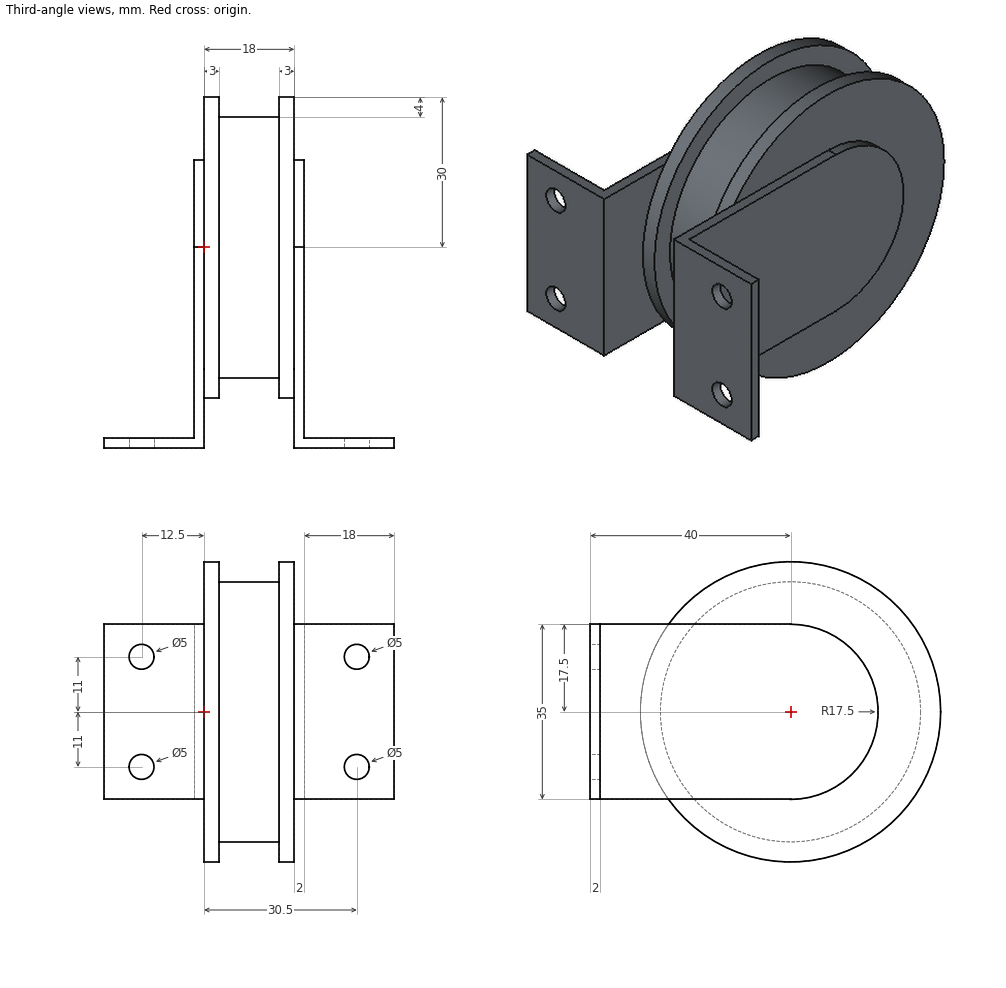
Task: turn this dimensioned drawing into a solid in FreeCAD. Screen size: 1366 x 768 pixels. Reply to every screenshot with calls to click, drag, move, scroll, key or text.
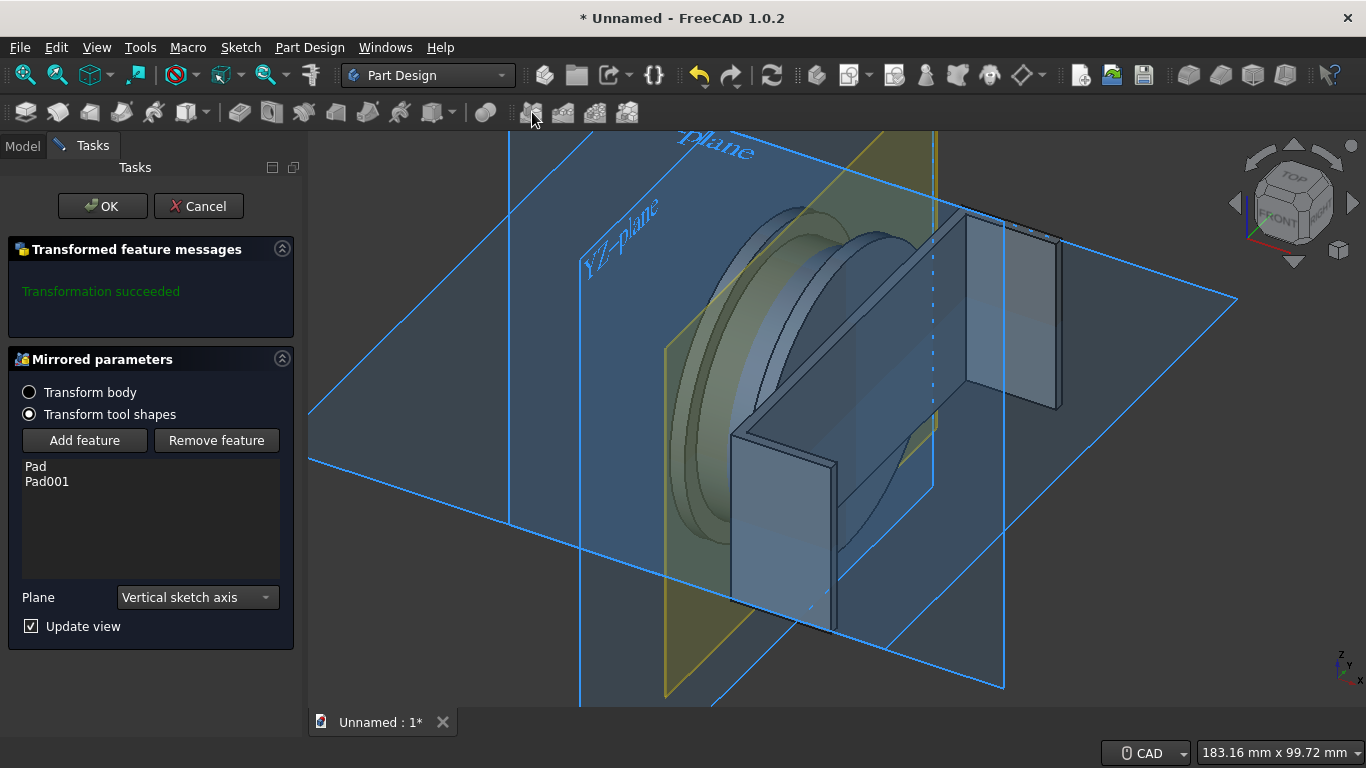
click(198, 598)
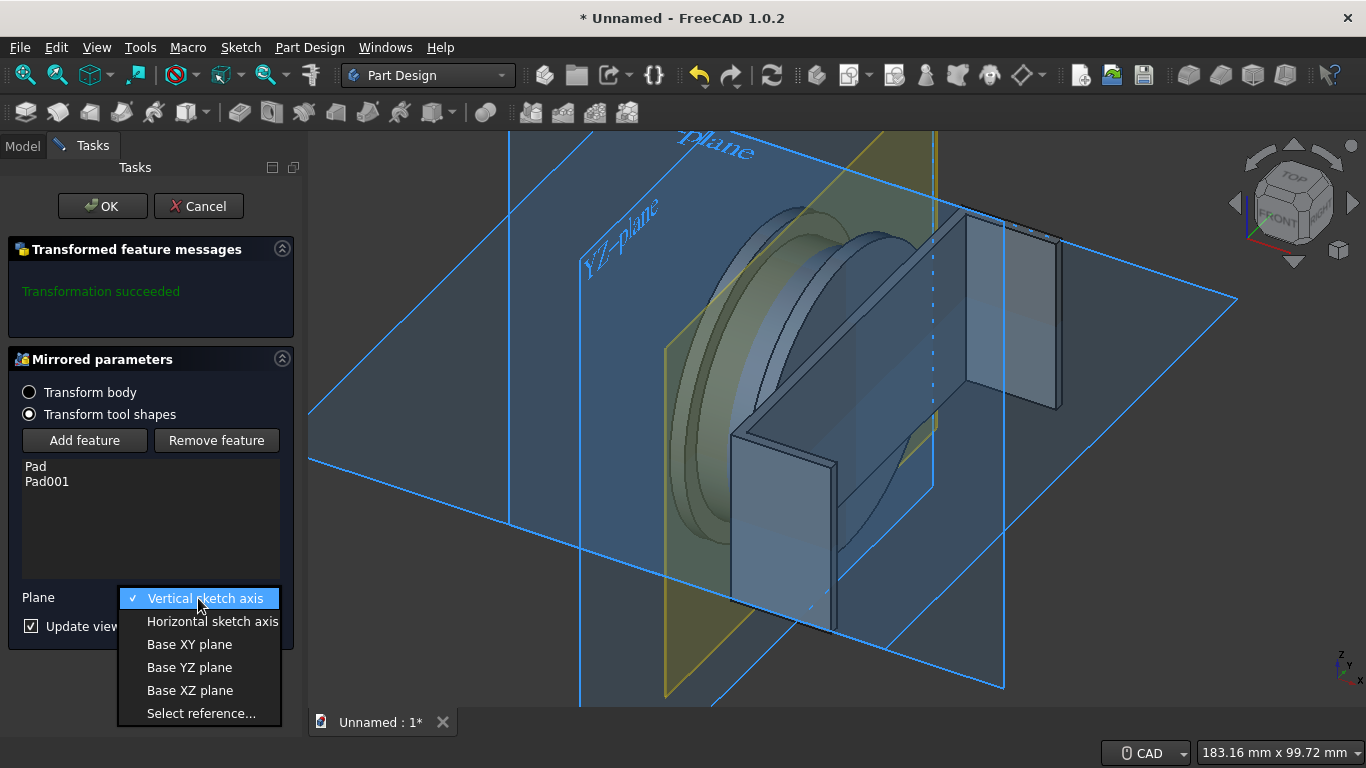
click(198, 714)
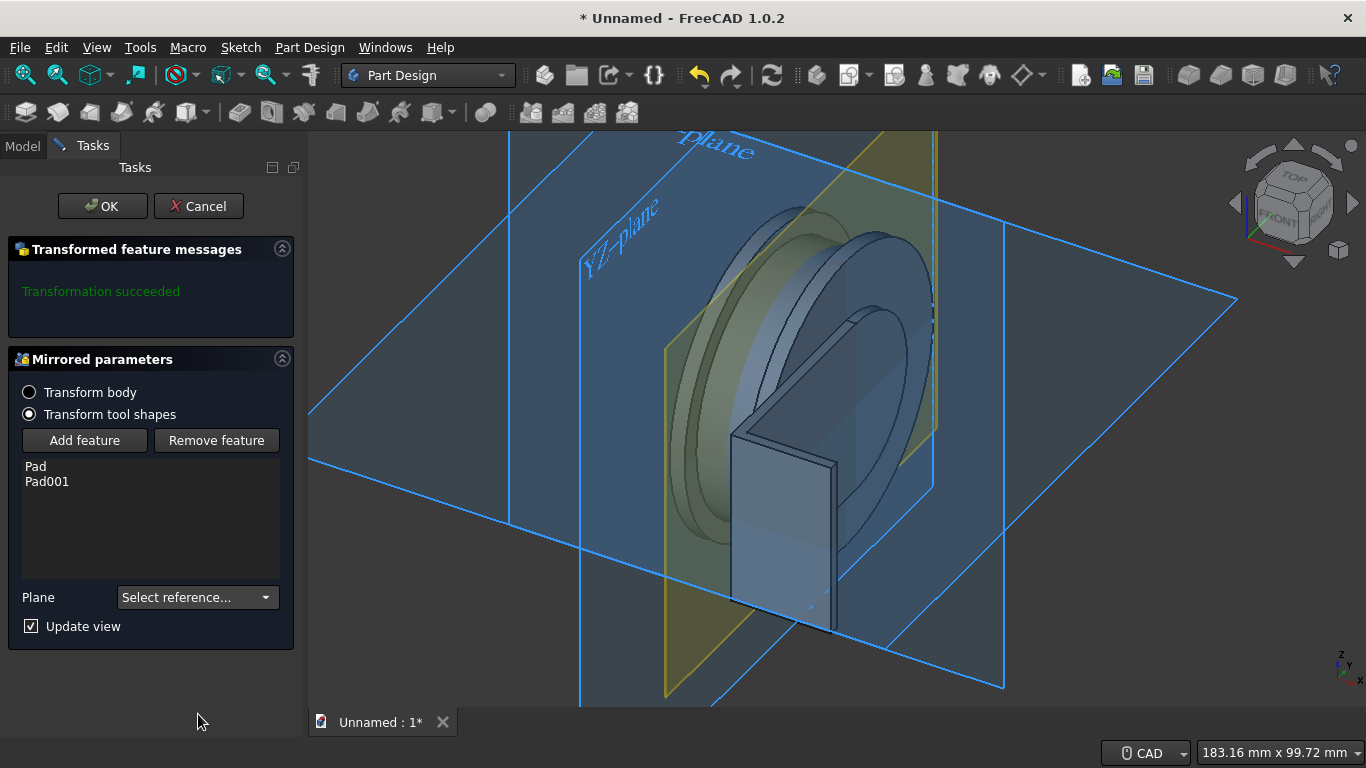
click(23, 145)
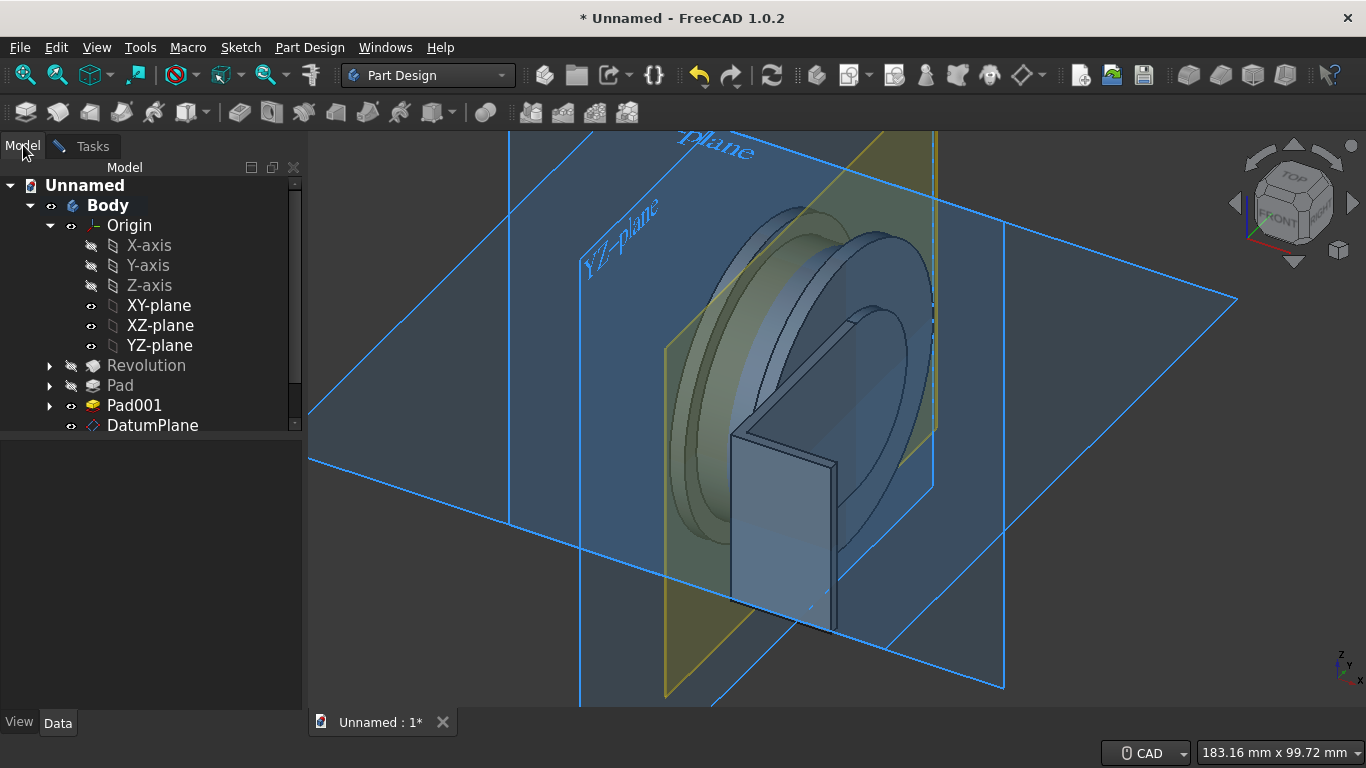
click(116, 426)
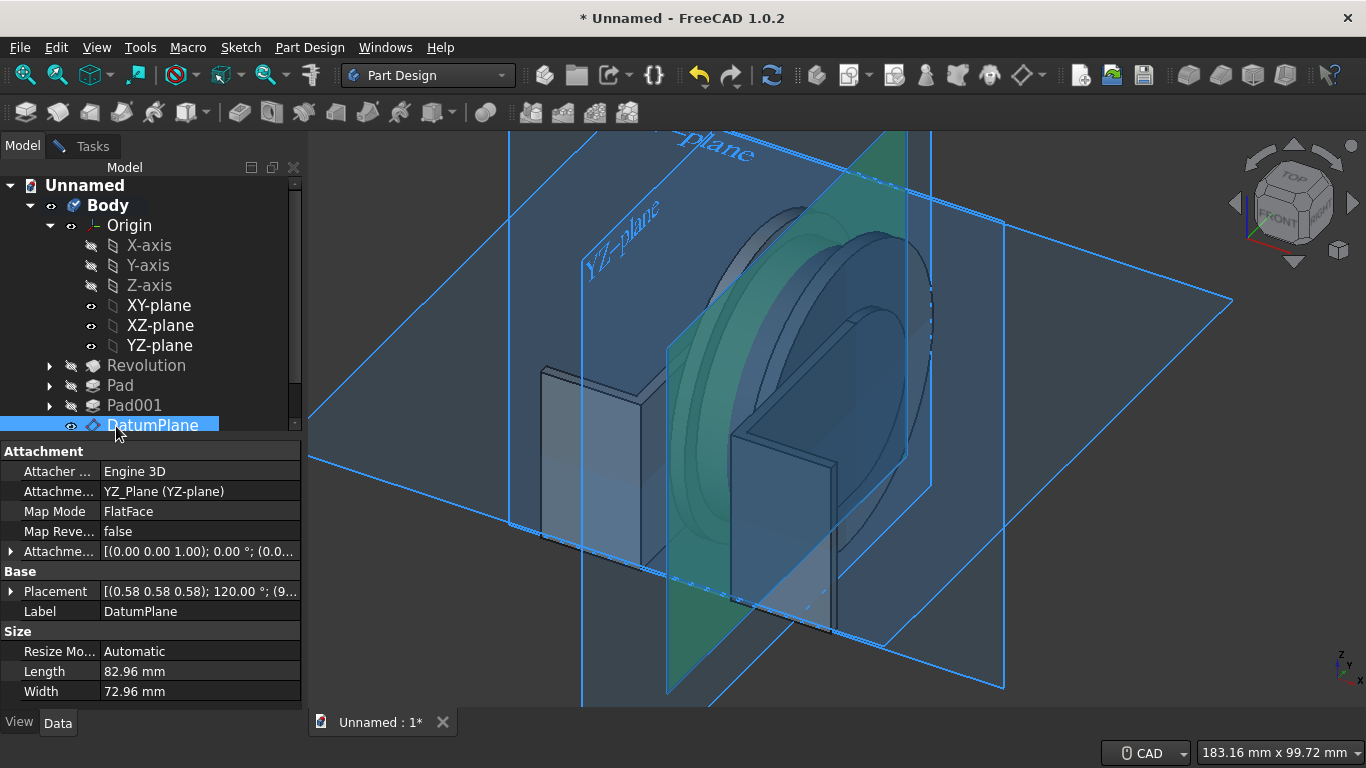
click(84, 145)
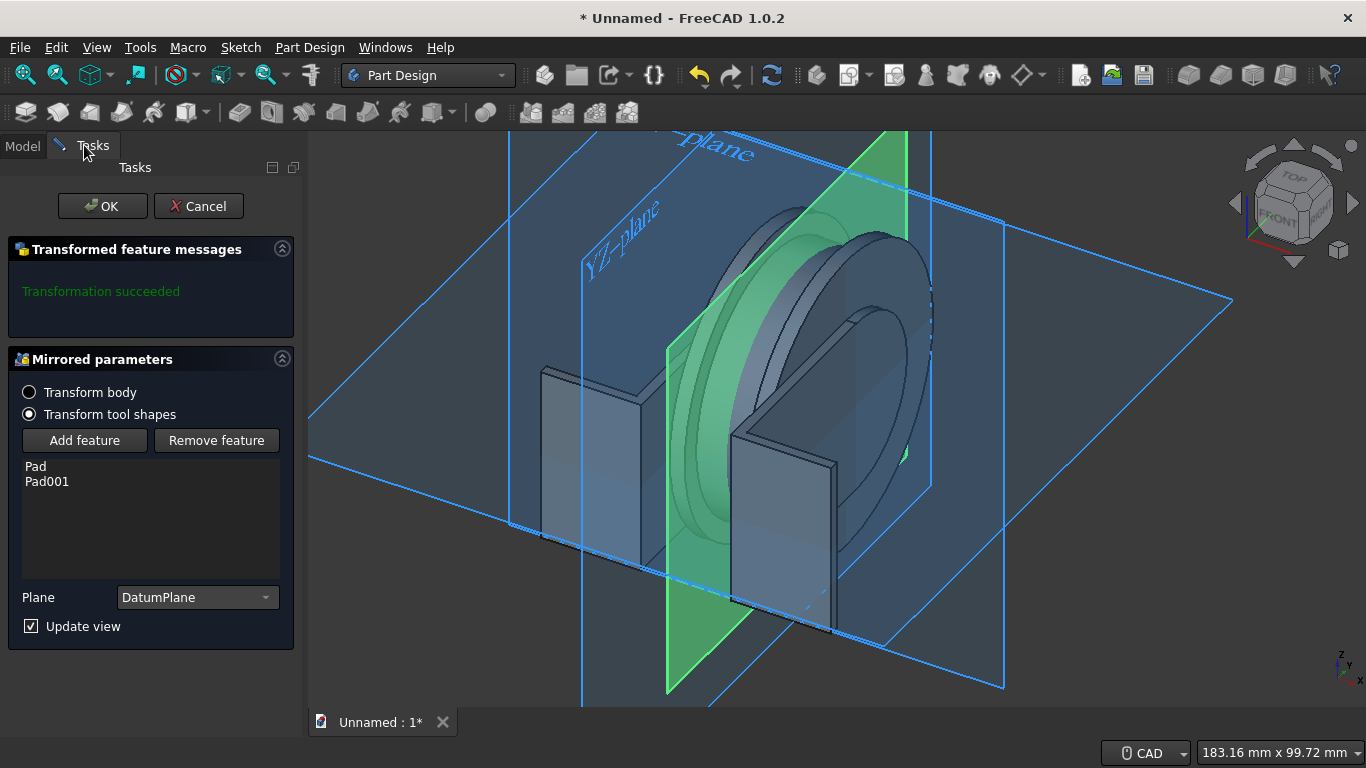
click(103, 206)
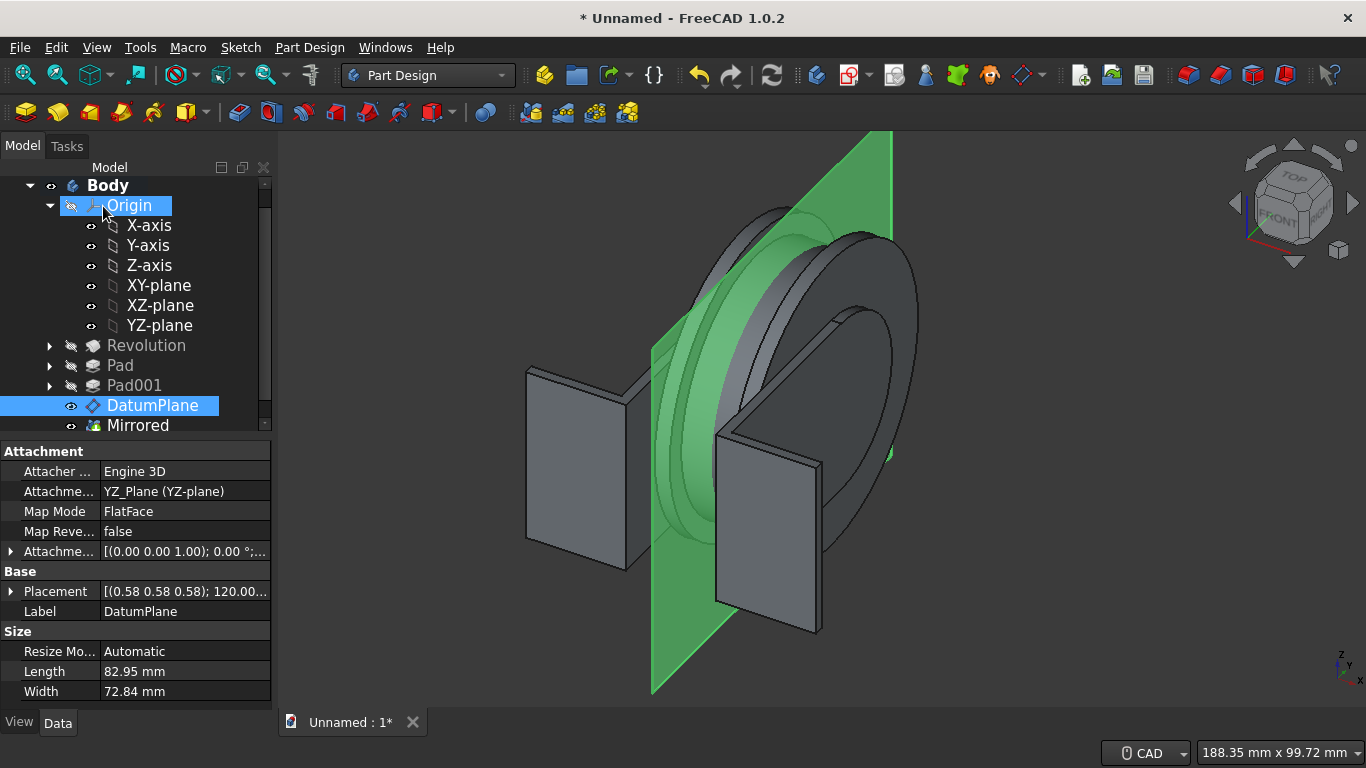
click(116, 406)
key(space)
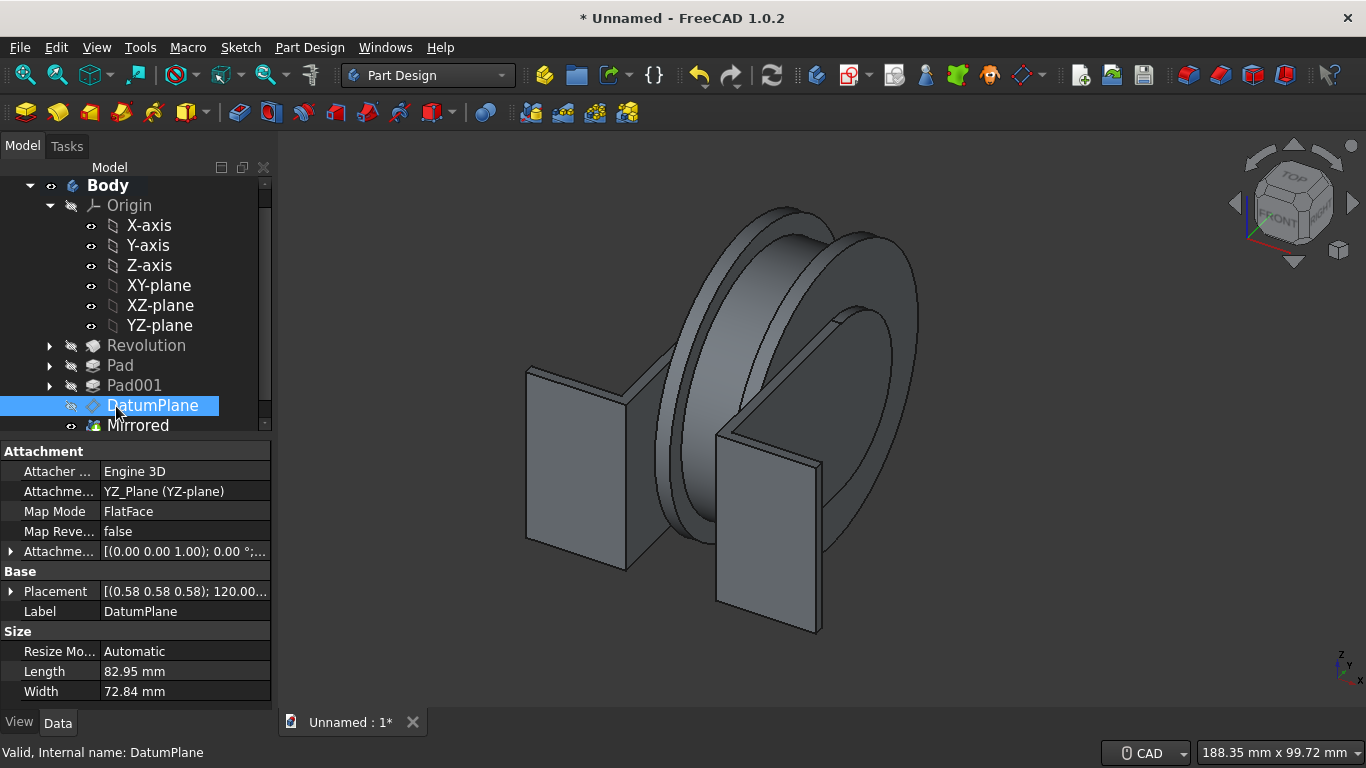
key(v)
key(f)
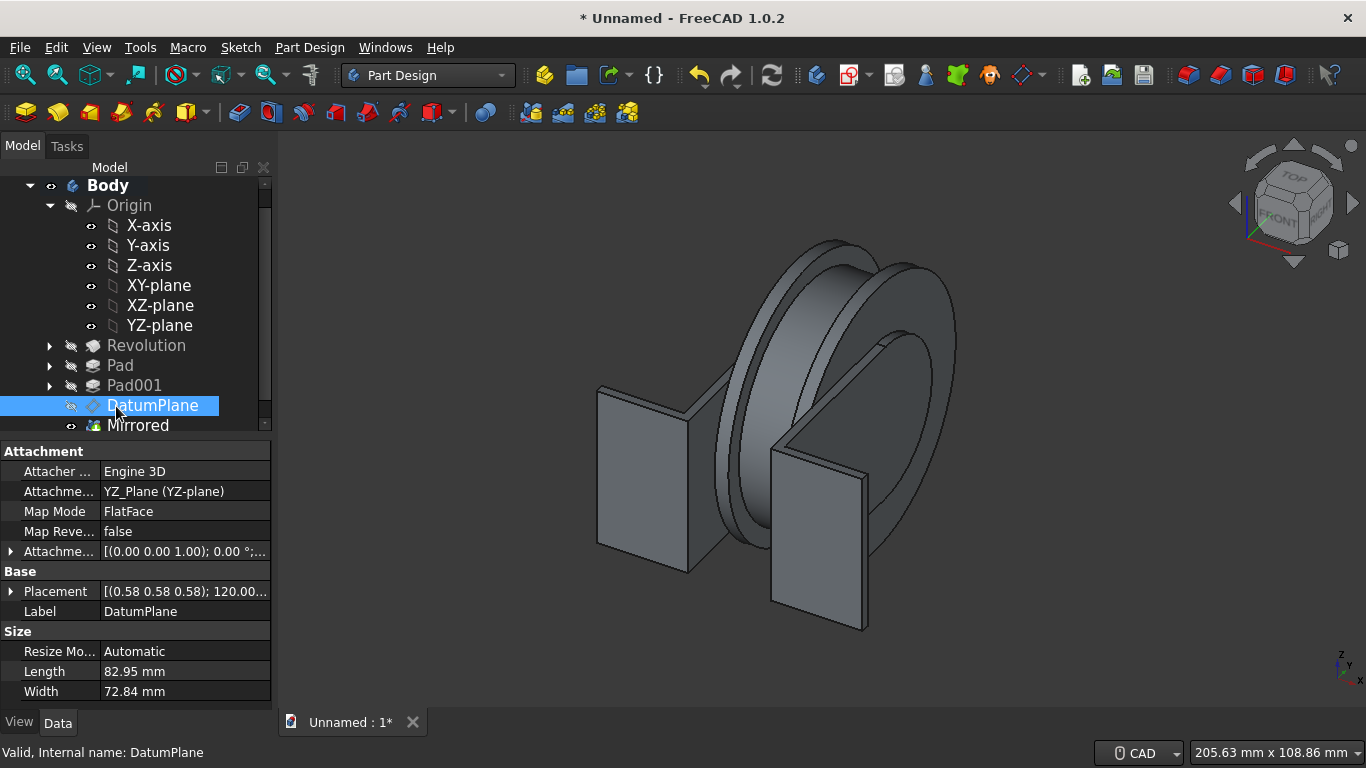
click(816, 517)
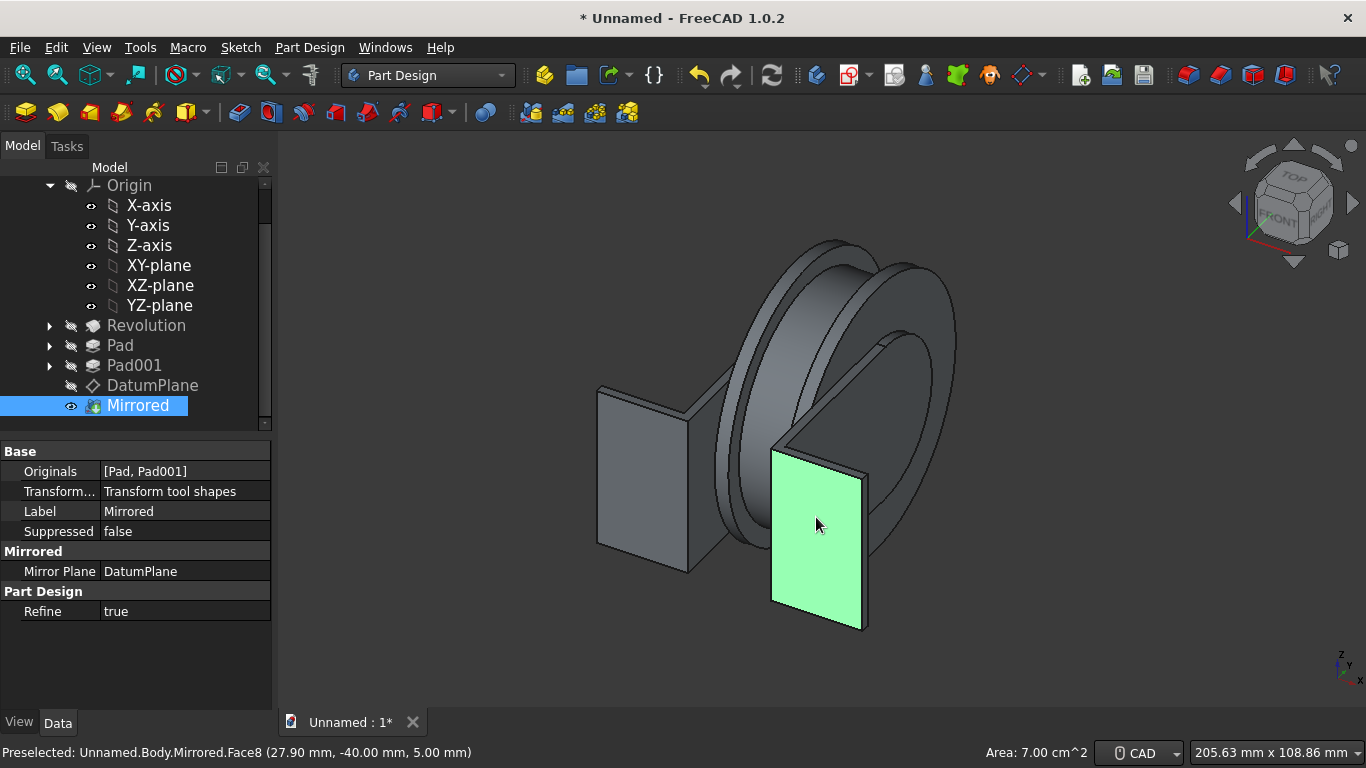
click(850, 76)